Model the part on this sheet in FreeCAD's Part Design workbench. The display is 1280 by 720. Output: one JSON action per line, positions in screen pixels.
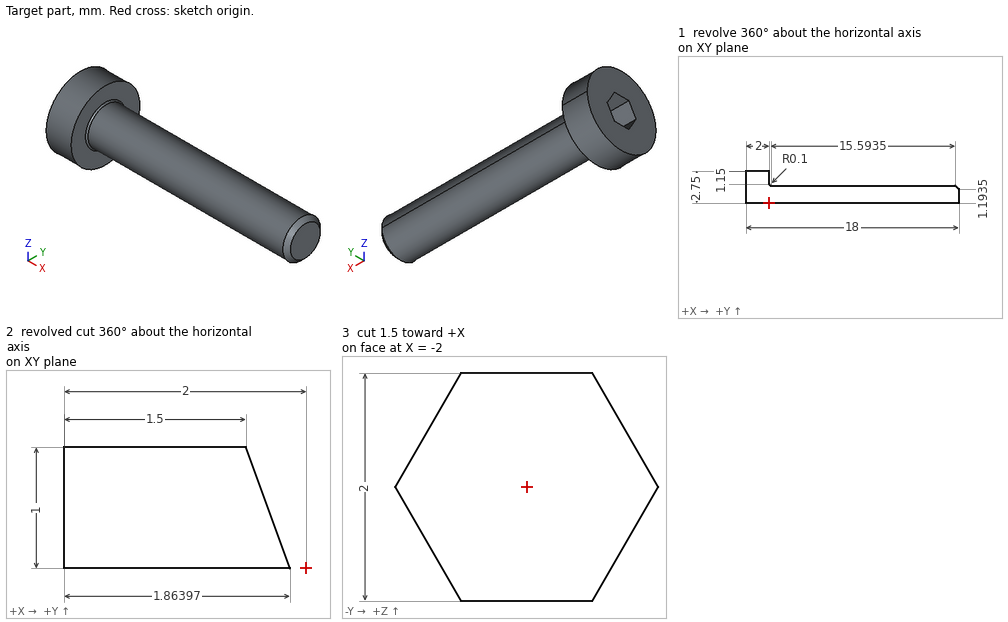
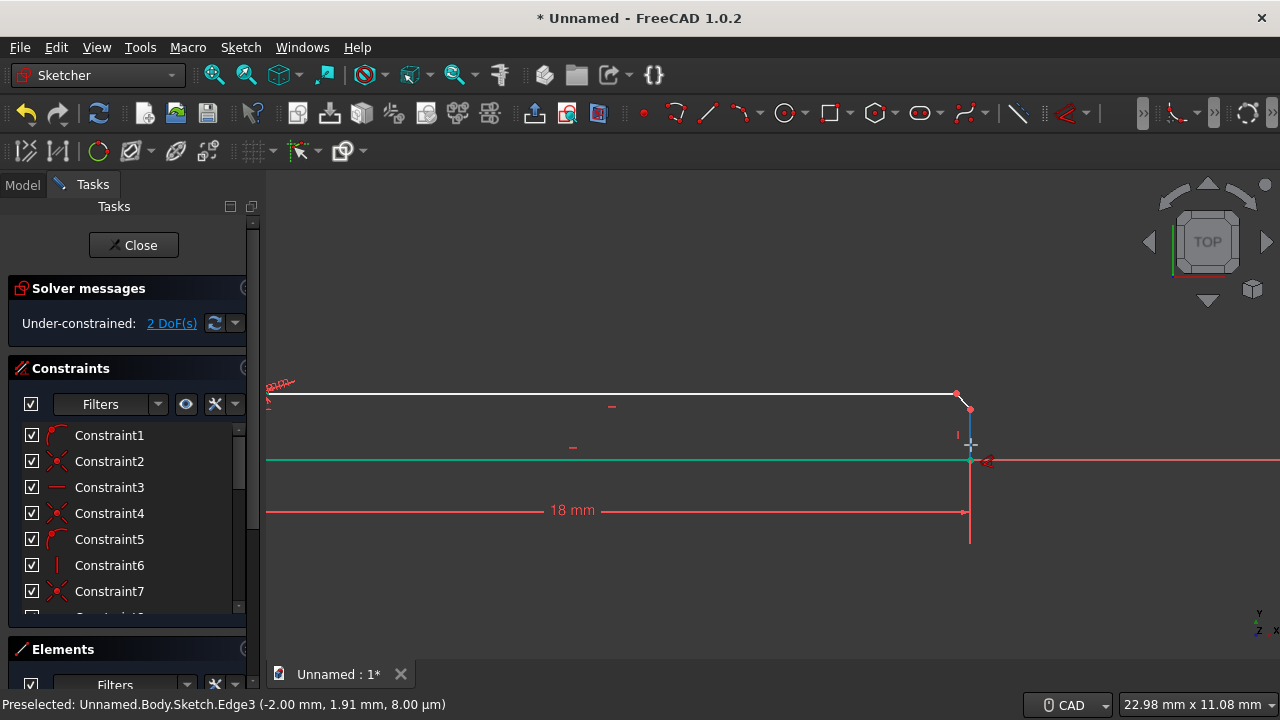
{"action": "left_click", "coordinate": [970, 445]}
{"action": "left_click", "coordinate": [1004, 435]}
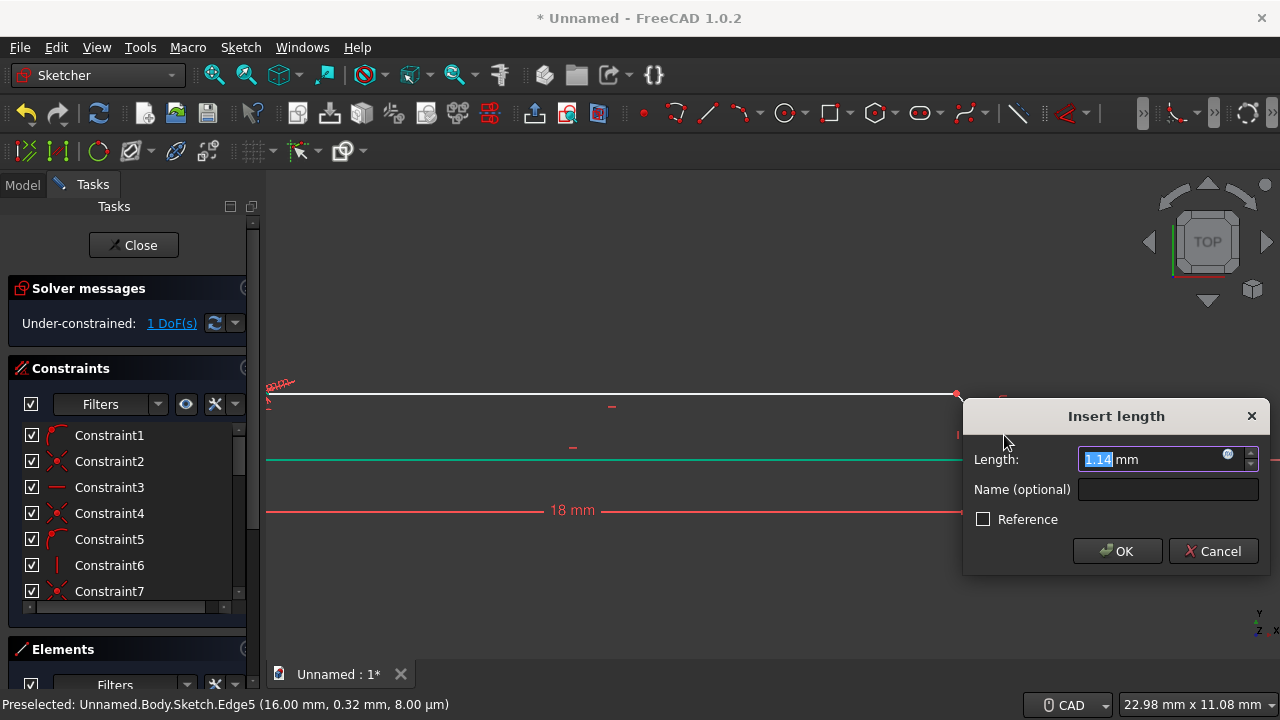
{"action": "type", "text": "1.1935"}
{"action": "key", "text": "Return"}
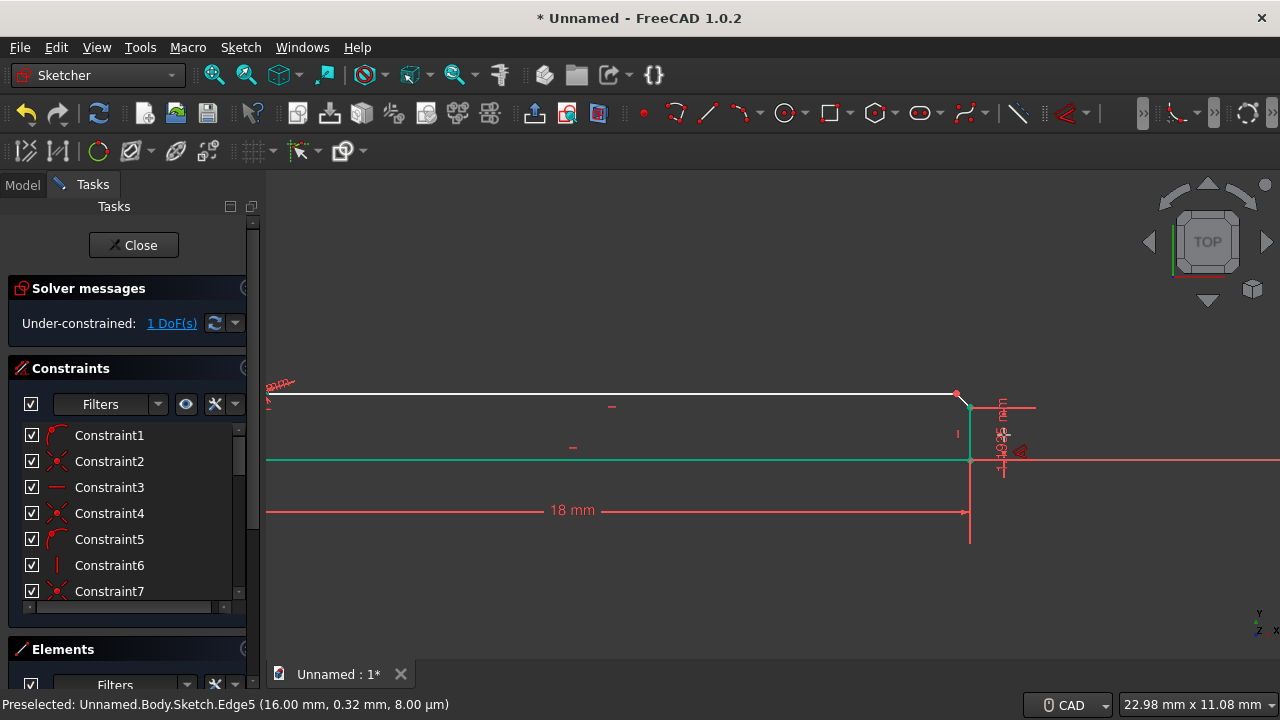
{"action": "left_click", "coordinate": [750, 394]}
{"action": "left_click", "coordinate": [625, 360]}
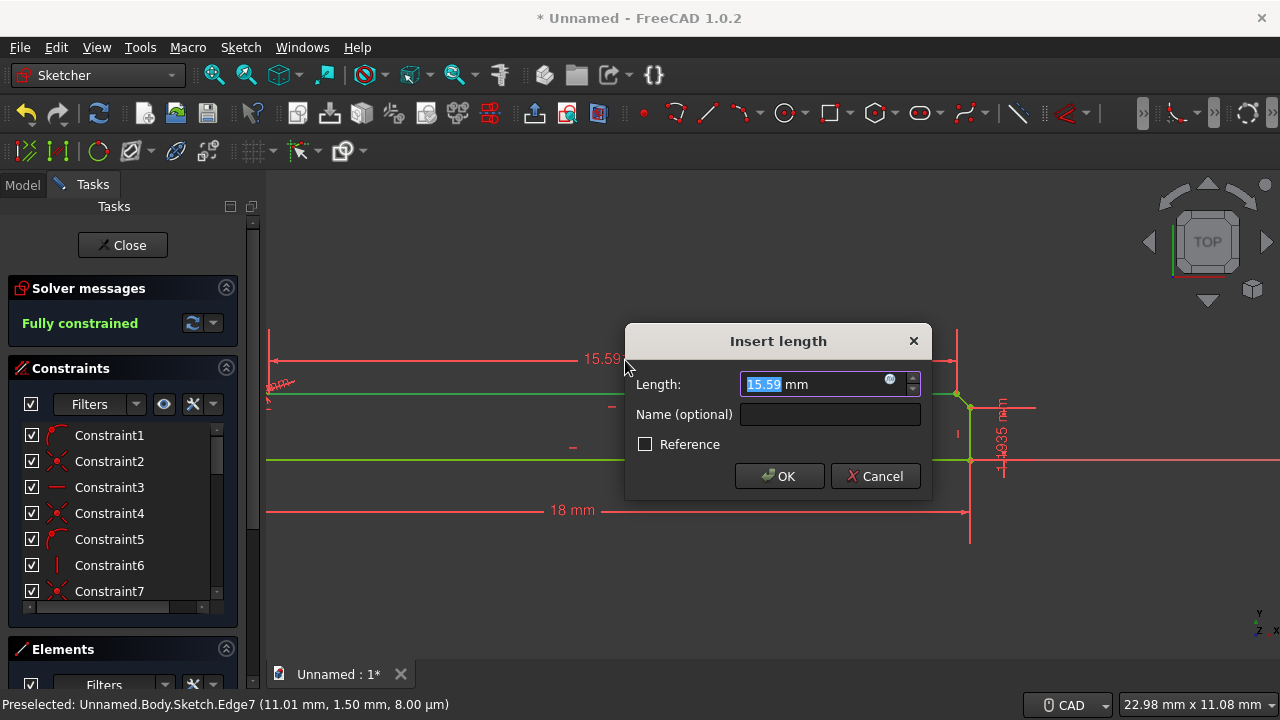
{"action": "type", "text": "15.5935"}
{"action": "key", "text": "Return"}
{"action": "key", "text": "Escape"}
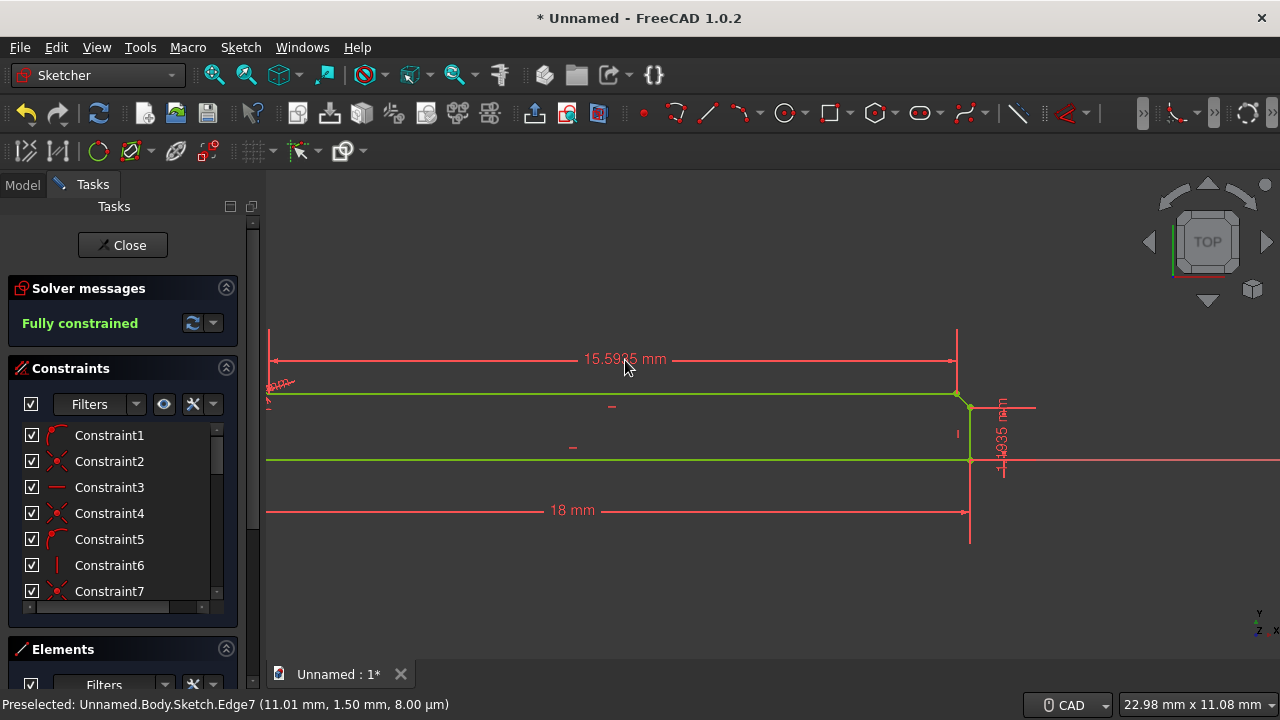
{"action": "left_click", "coordinate": [123, 245]}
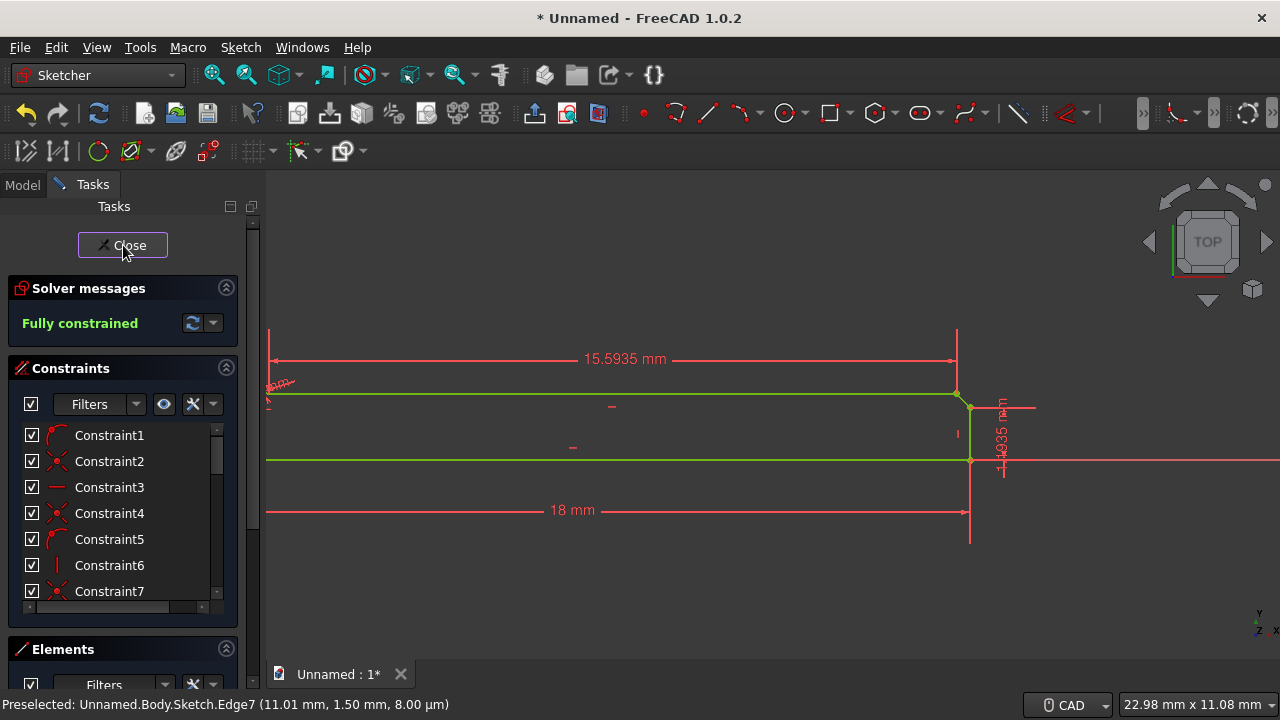
{"action": "left_click", "coordinate": [58, 76]}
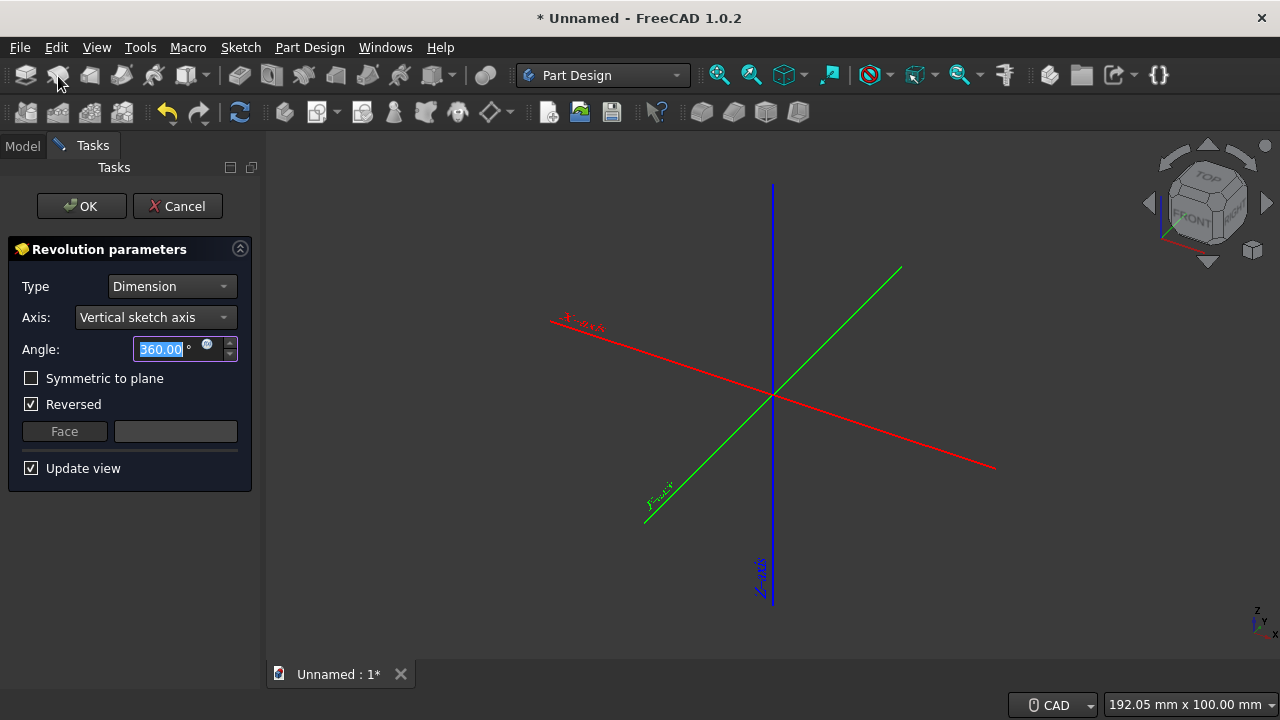
{"action": "left_click", "coordinate": [156, 318]}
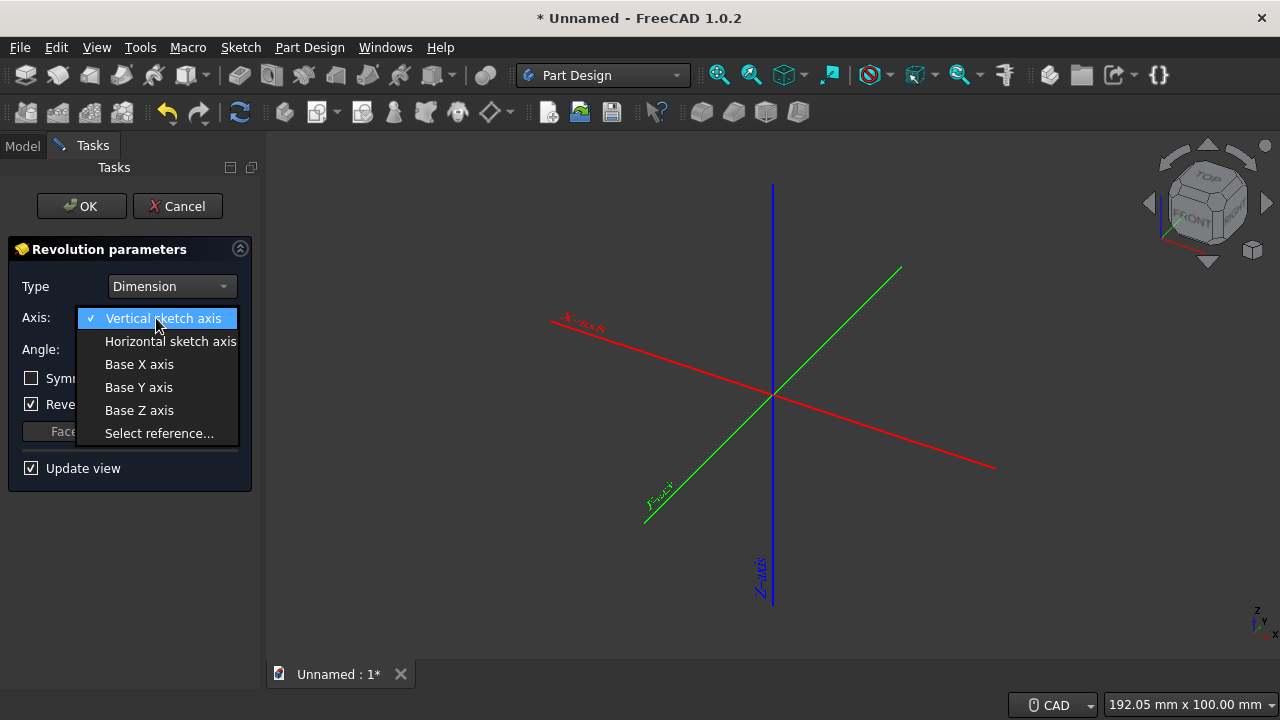
{"action": "left_click", "coordinate": [156, 342]}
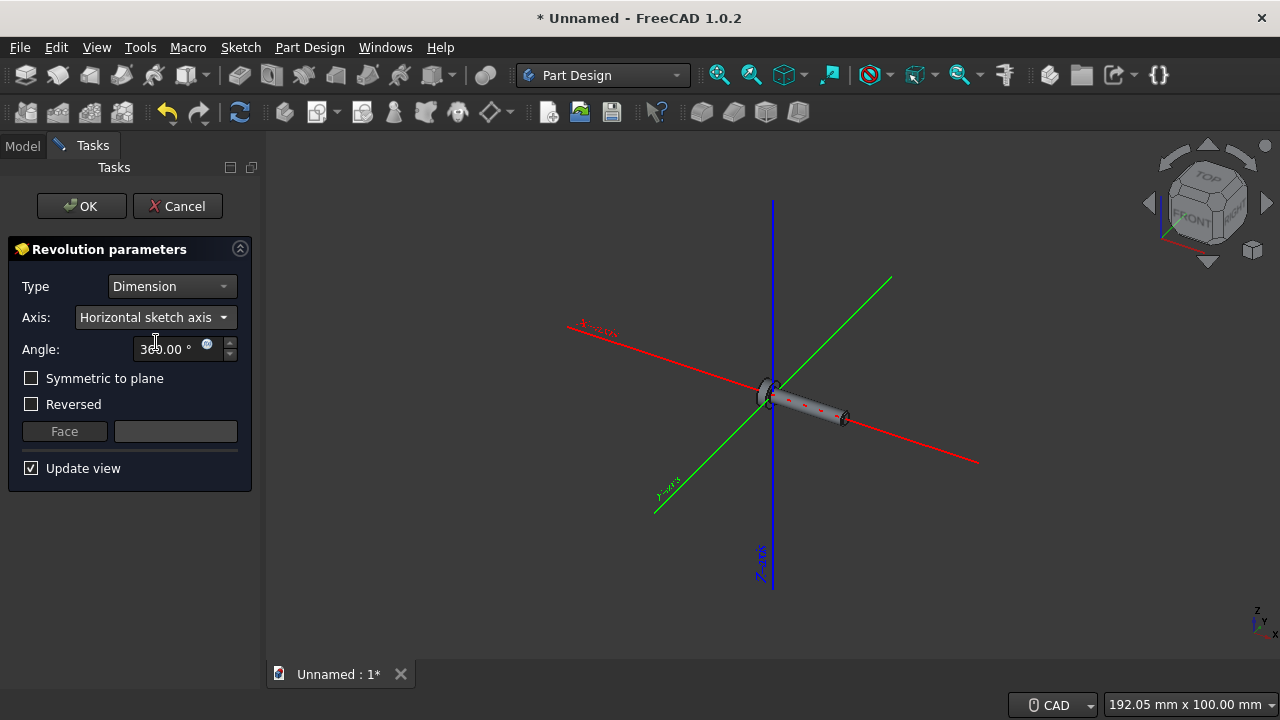
{"action": "left_click", "coordinate": [82, 206]}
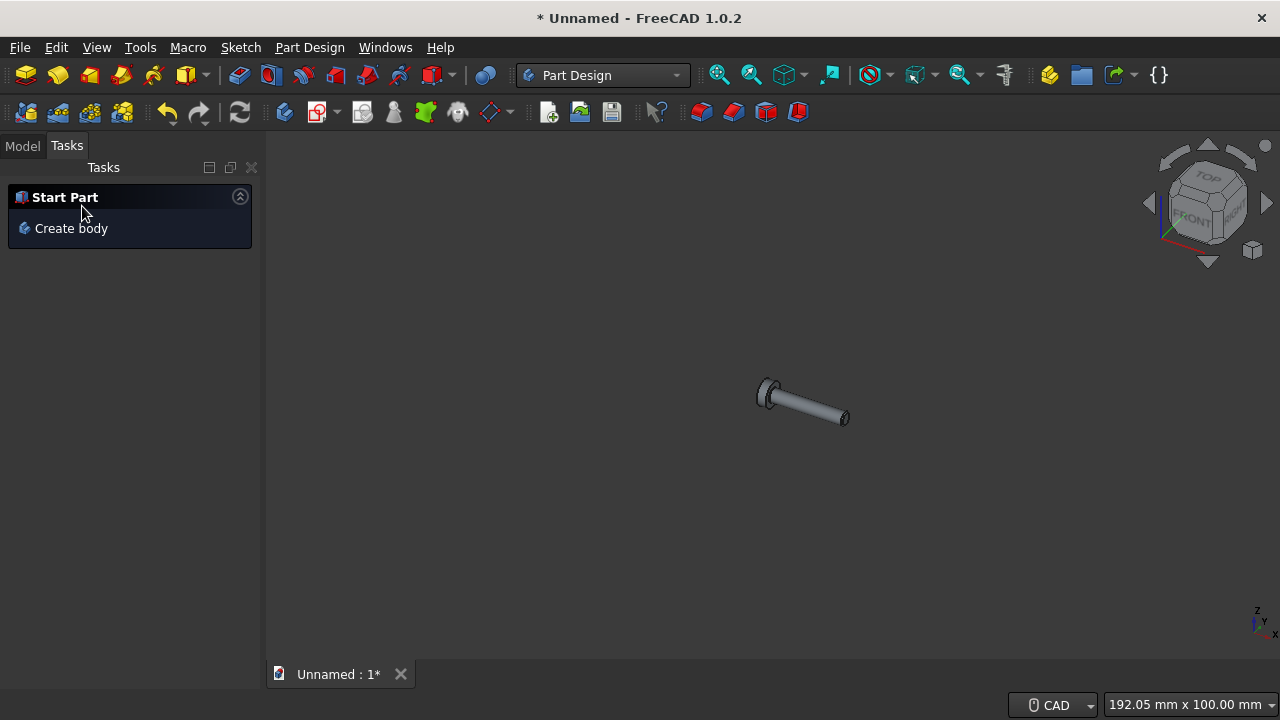
{"action": "left_click", "coordinate": [720, 76]}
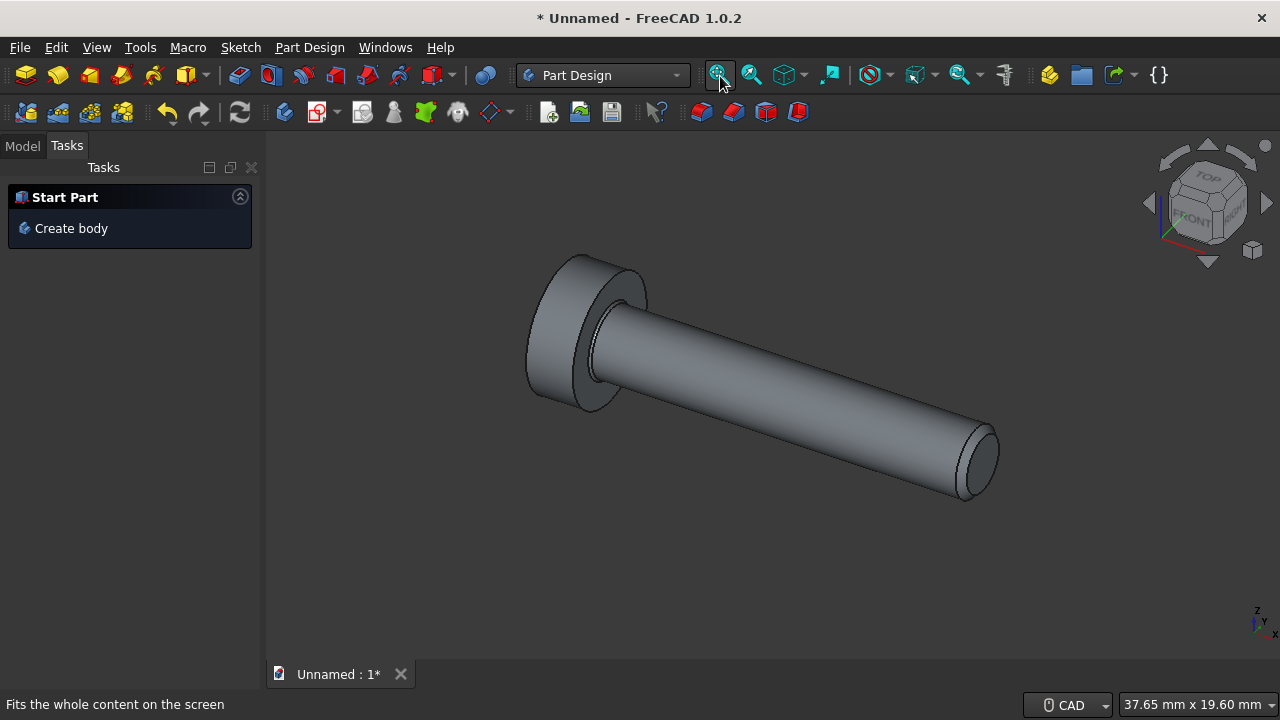
{"action": "left_click", "coordinate": [318, 112]}